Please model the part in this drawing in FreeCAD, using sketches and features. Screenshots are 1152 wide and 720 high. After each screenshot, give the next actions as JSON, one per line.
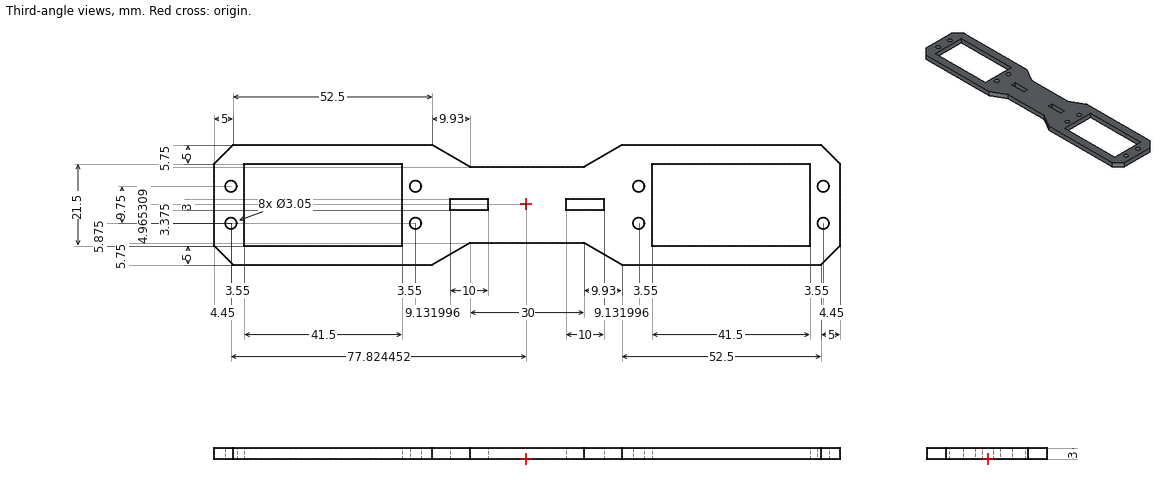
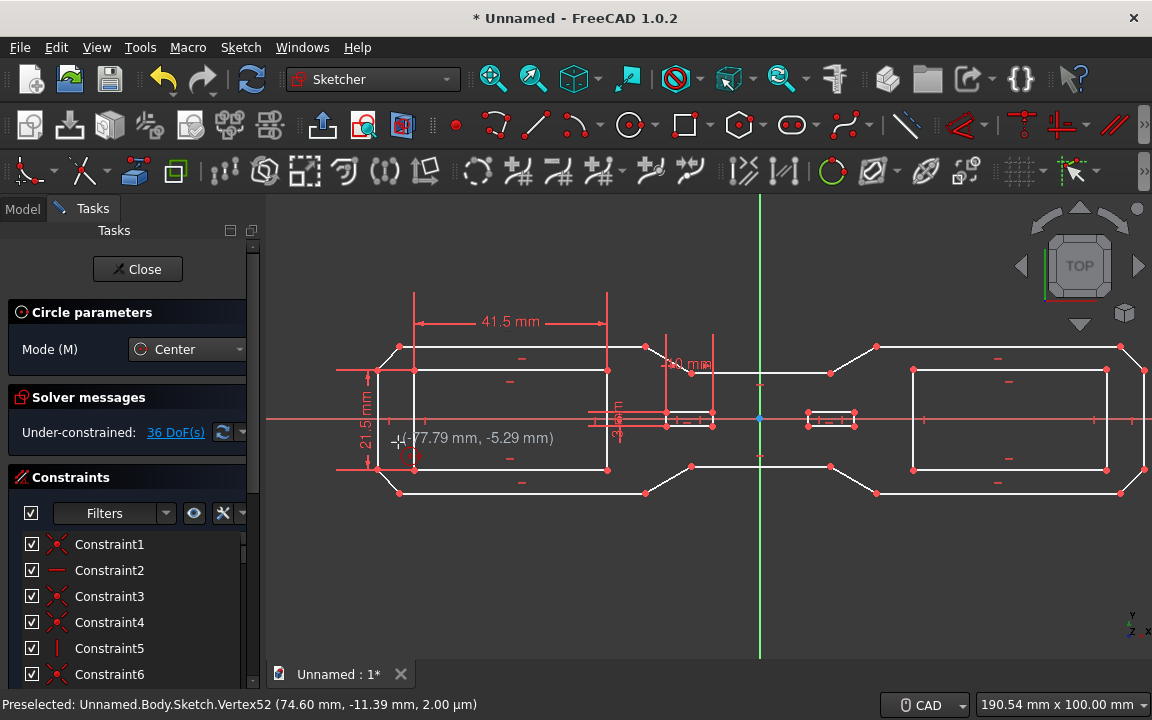
{"action": "left_click", "coordinate": [398, 442]}
{"action": "mouse_move", "coordinate": [393, 437]}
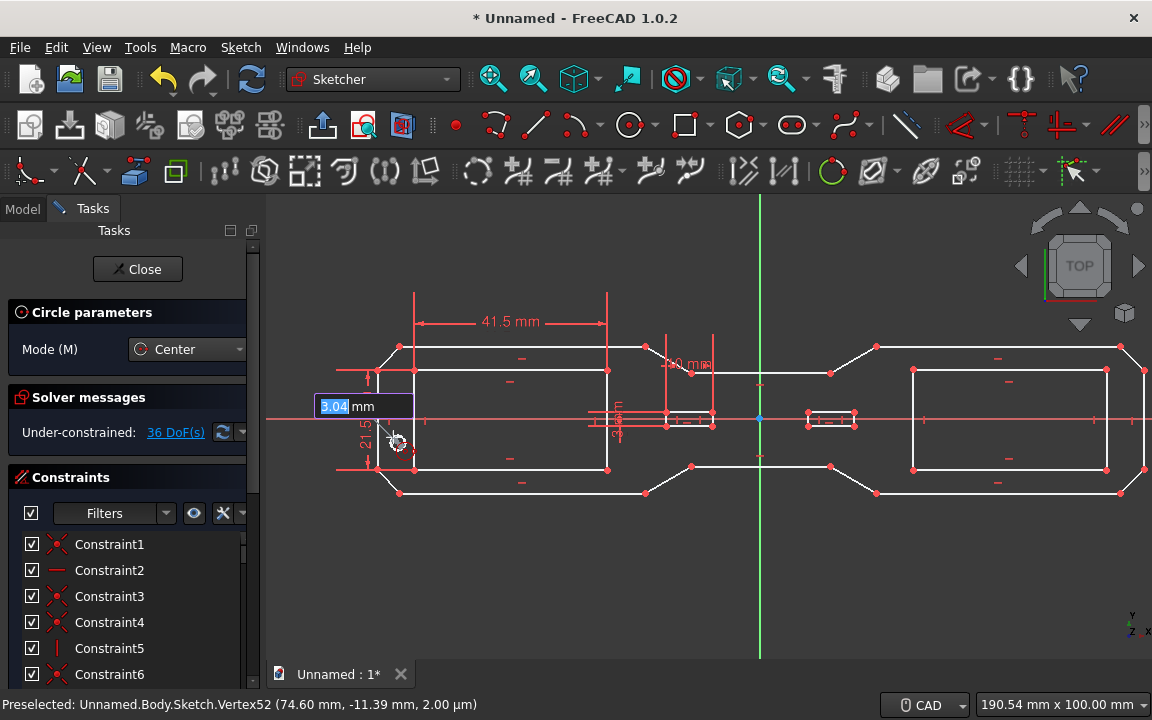
{"action": "type", "text": "3.05"}
{"action": "key", "text": "Return"}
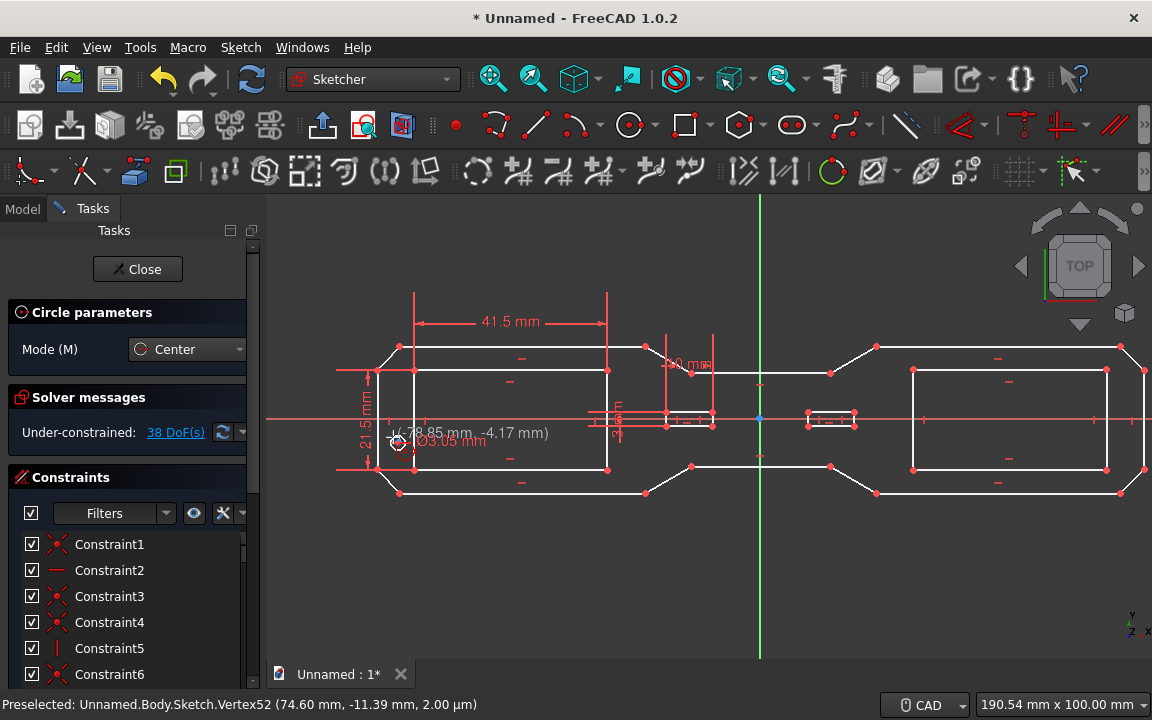
{"action": "scroll", "coordinate": [624, 442], "scroll_direction": "up", "scroll_amount": 6}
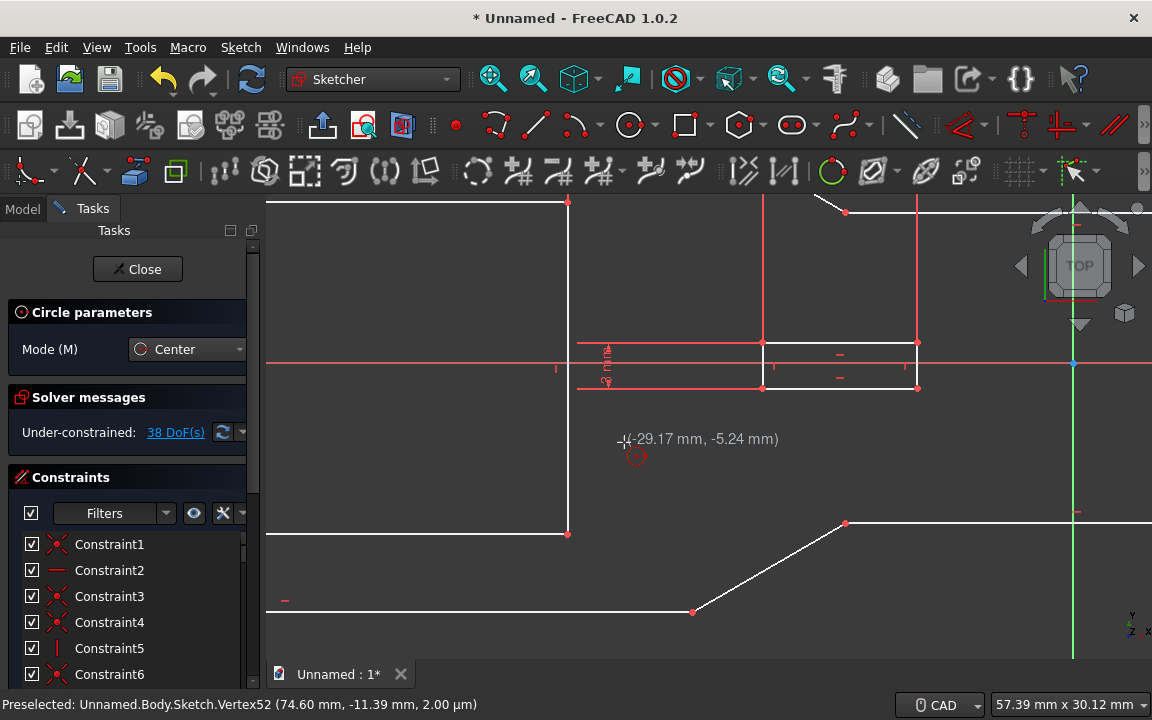
{"action": "scroll", "coordinate": [530, 442], "scroll_direction": "down", "scroll_amount": 8}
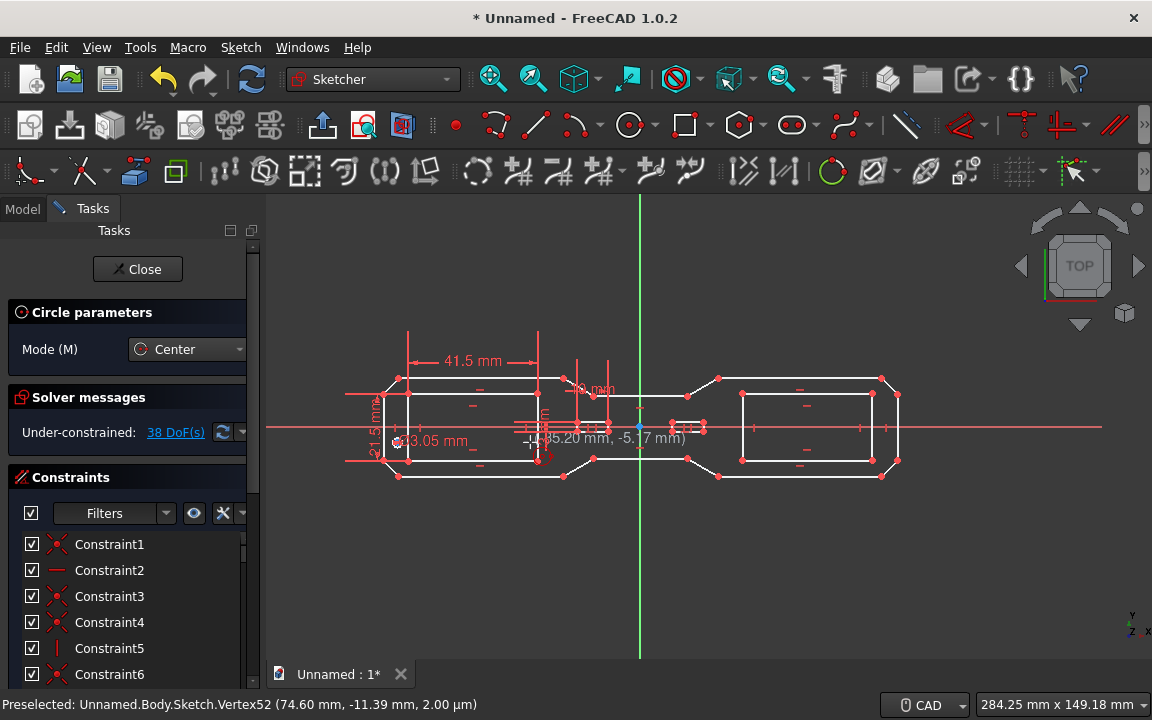
{"action": "scroll", "coordinate": [549, 442], "scroll_direction": "up", "scroll_amount": 2}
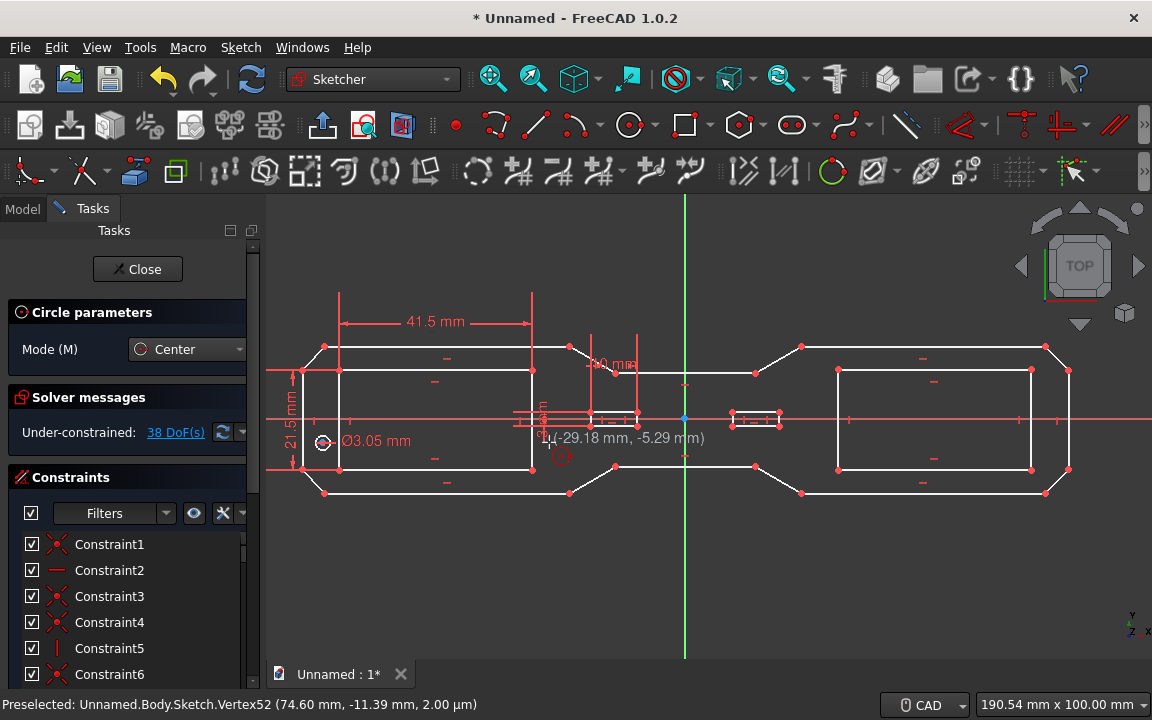
{"action": "left_click", "coordinate": [549, 442]}
{"action": "mouse_move", "coordinate": [554, 437]}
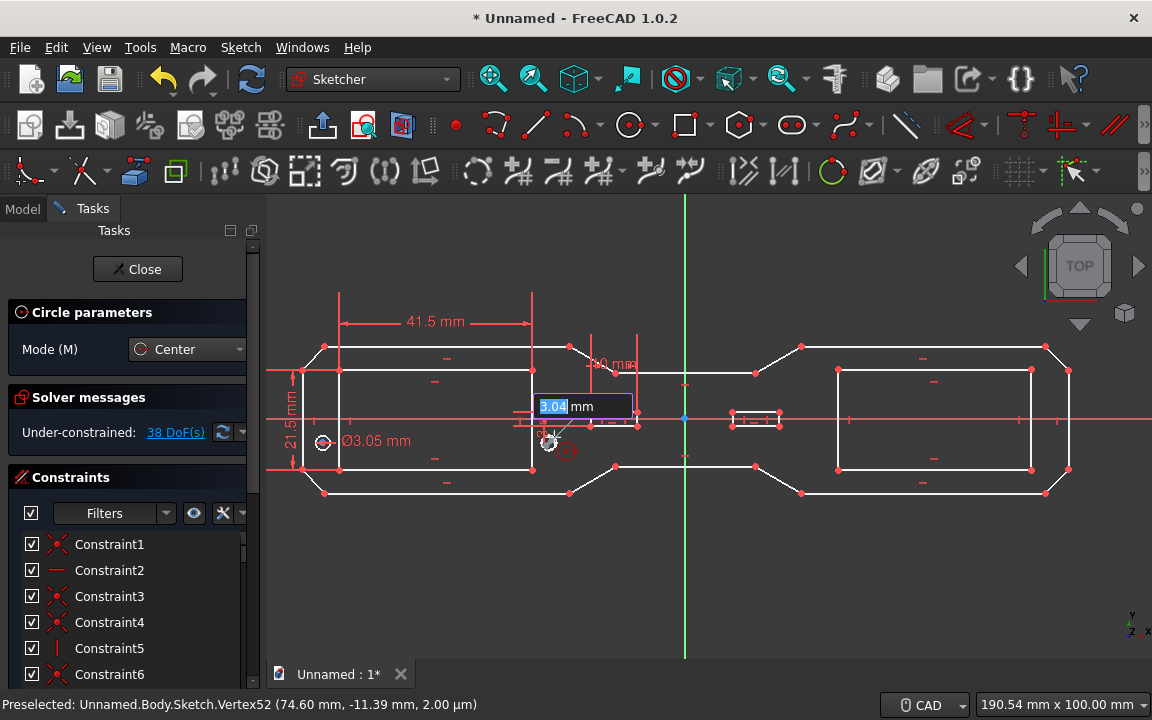
{"action": "type", "text": "3.05"}
{"action": "key", "text": "Return"}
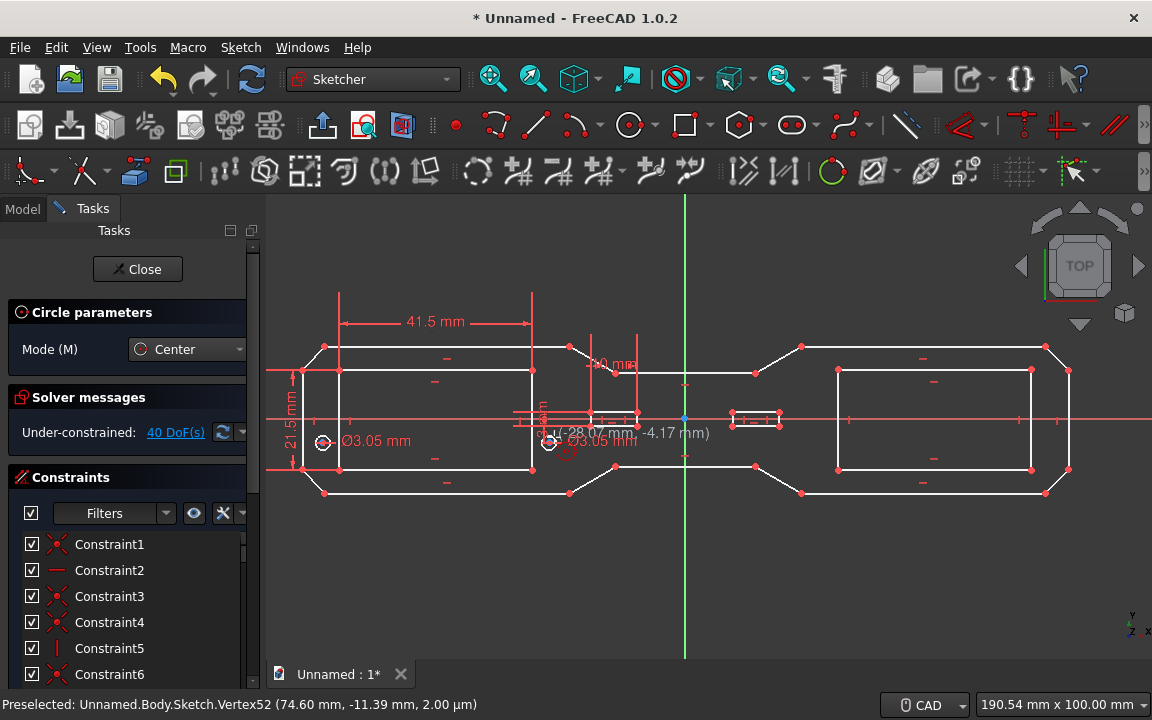
{"action": "scroll", "coordinate": [822, 442], "scroll_direction": "up", "scroll_amount": 6}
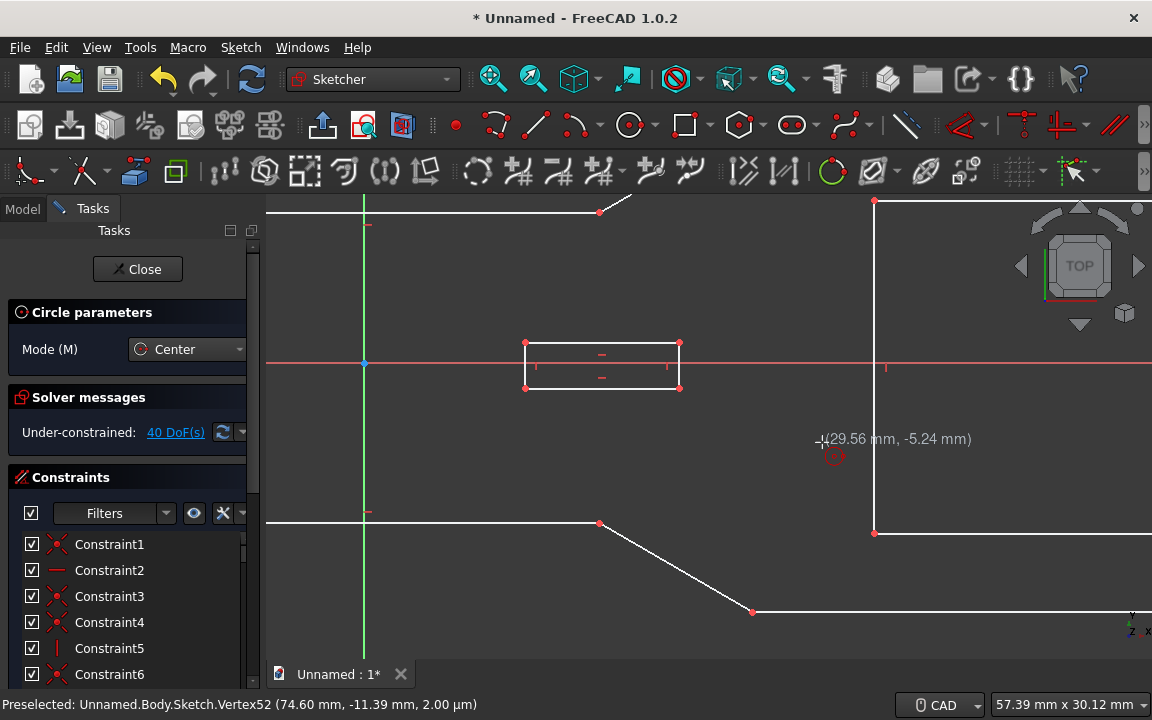
{"action": "scroll", "coordinate": [710, 442], "scroll_direction": "down", "scroll_amount": 8}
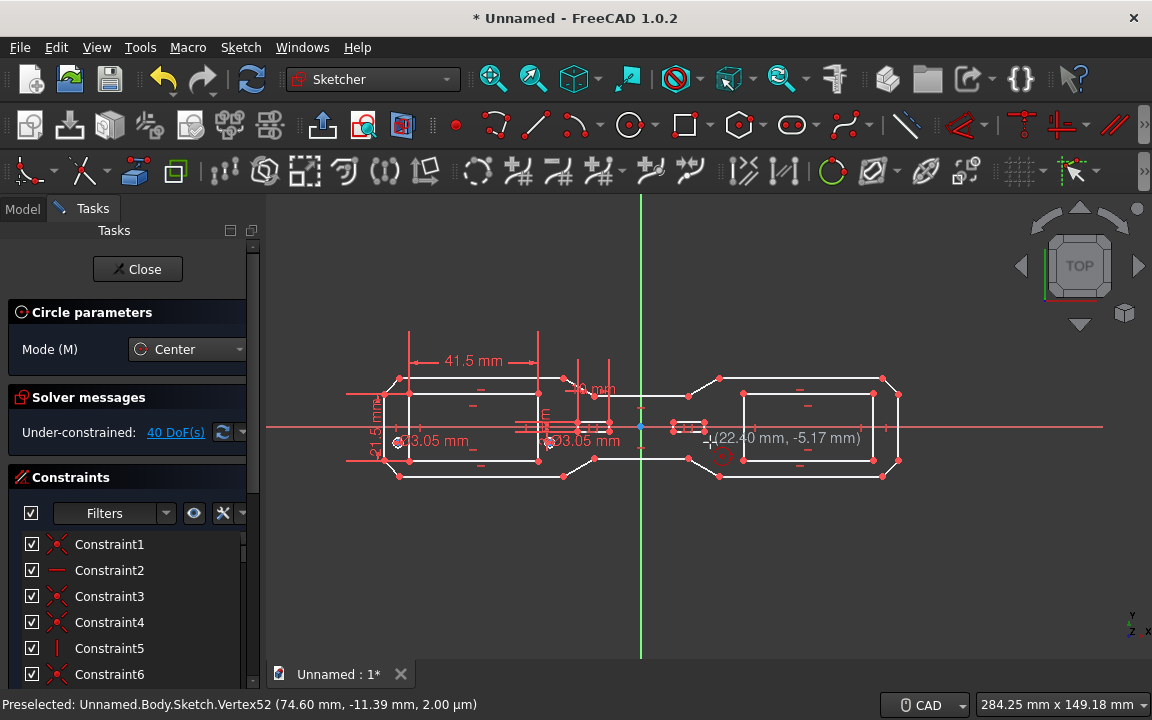
{"action": "scroll", "coordinate": [733, 442], "scroll_direction": "up", "scroll_amount": 2}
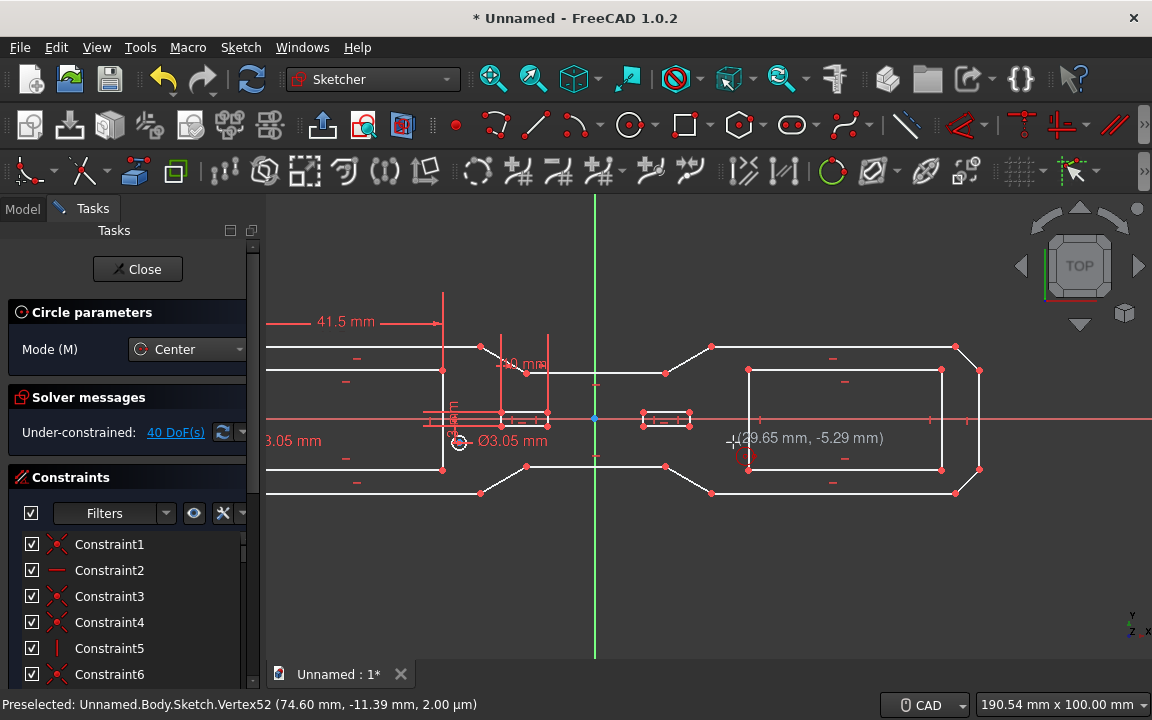
{"action": "left_click", "coordinate": [732, 442]}
{"action": "mouse_move", "coordinate": [727, 437]}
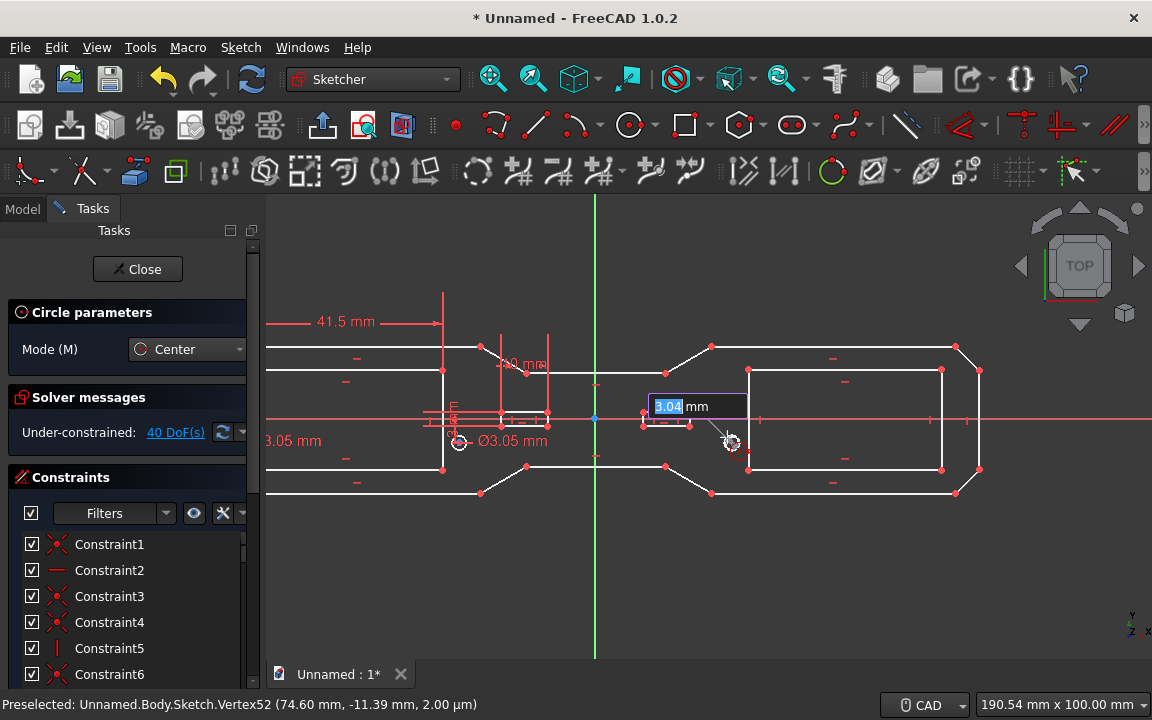
{"action": "type", "text": "3.05"}
{"action": "key", "text": "Return"}